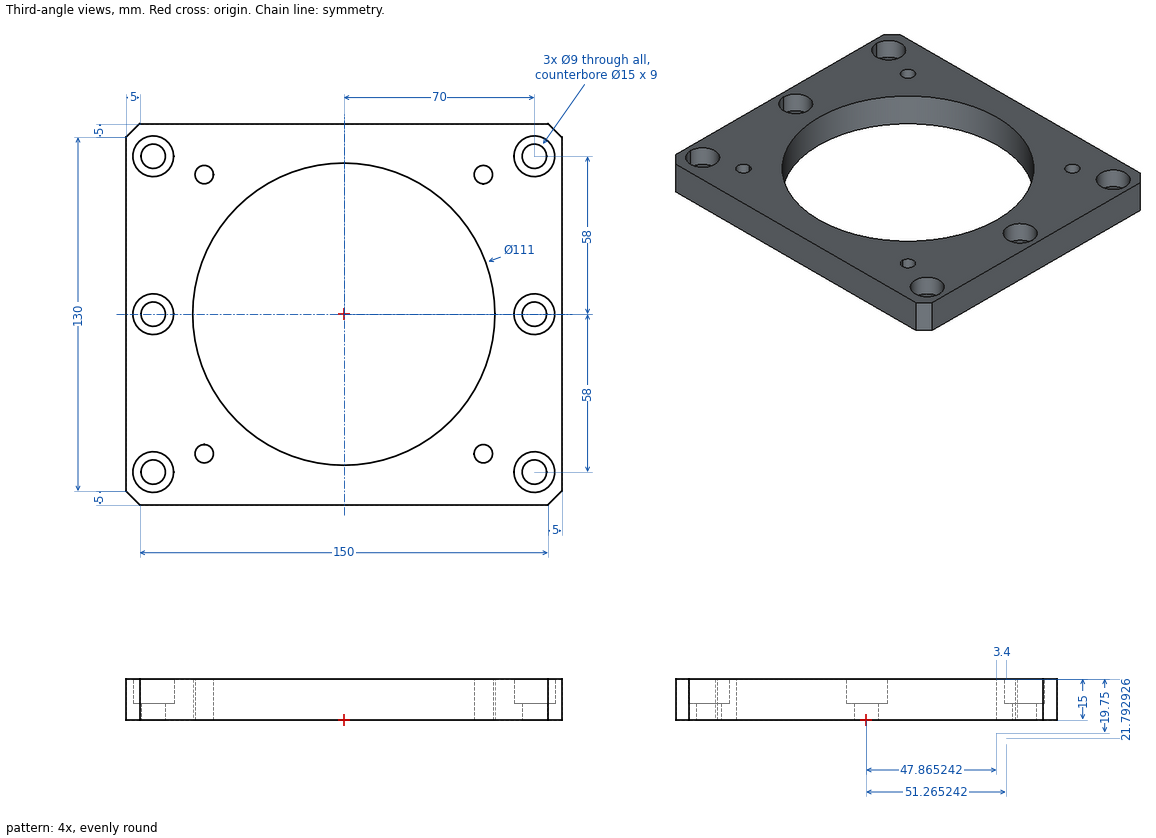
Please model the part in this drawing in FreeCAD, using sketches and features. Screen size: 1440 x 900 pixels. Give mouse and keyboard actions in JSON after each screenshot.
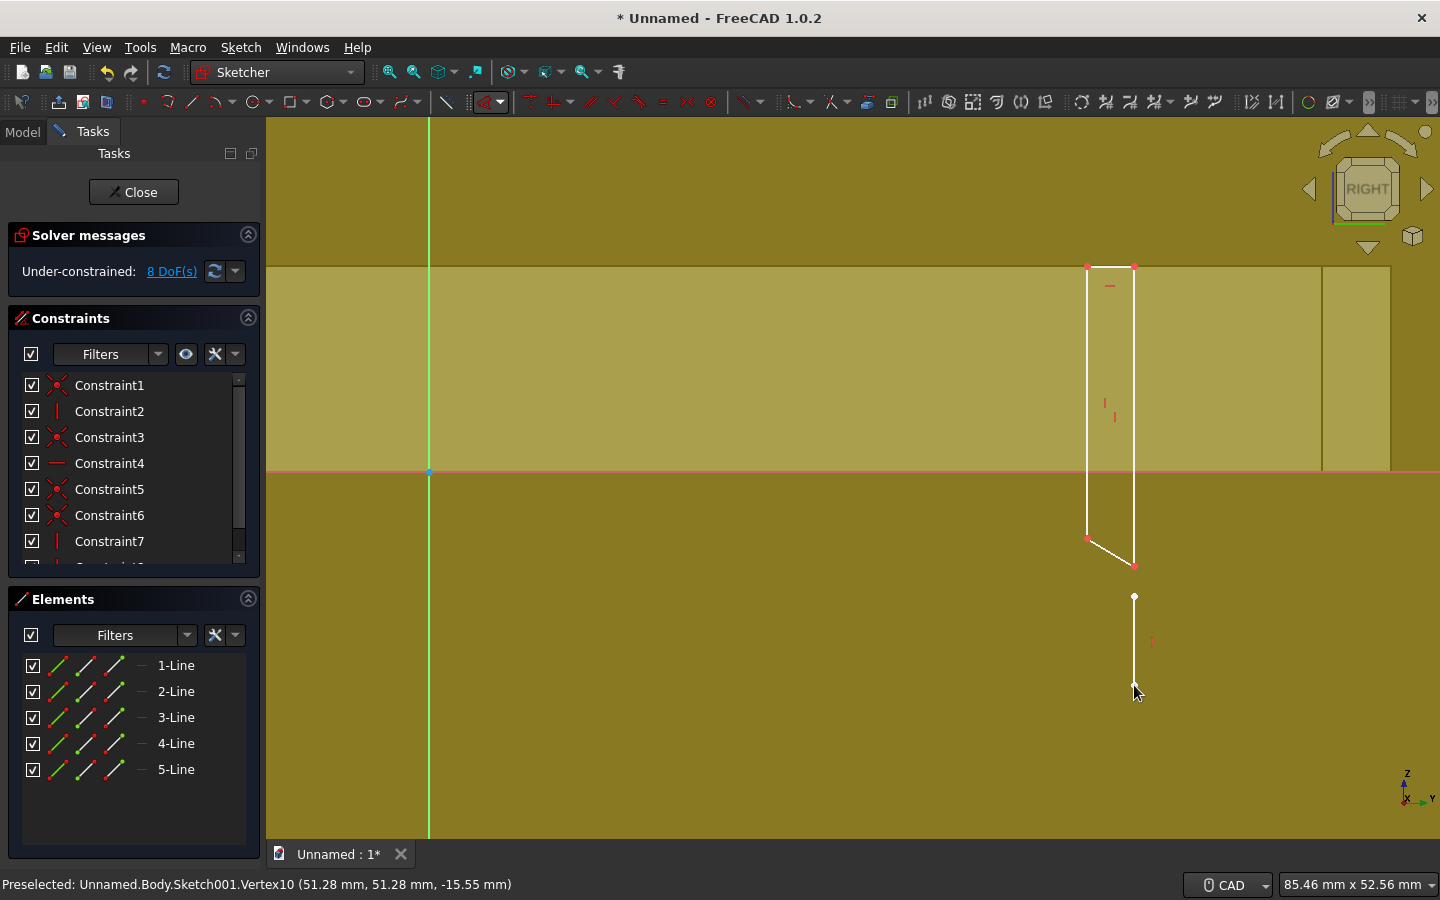
{"action": "left_click", "coordinate": [1134, 624]}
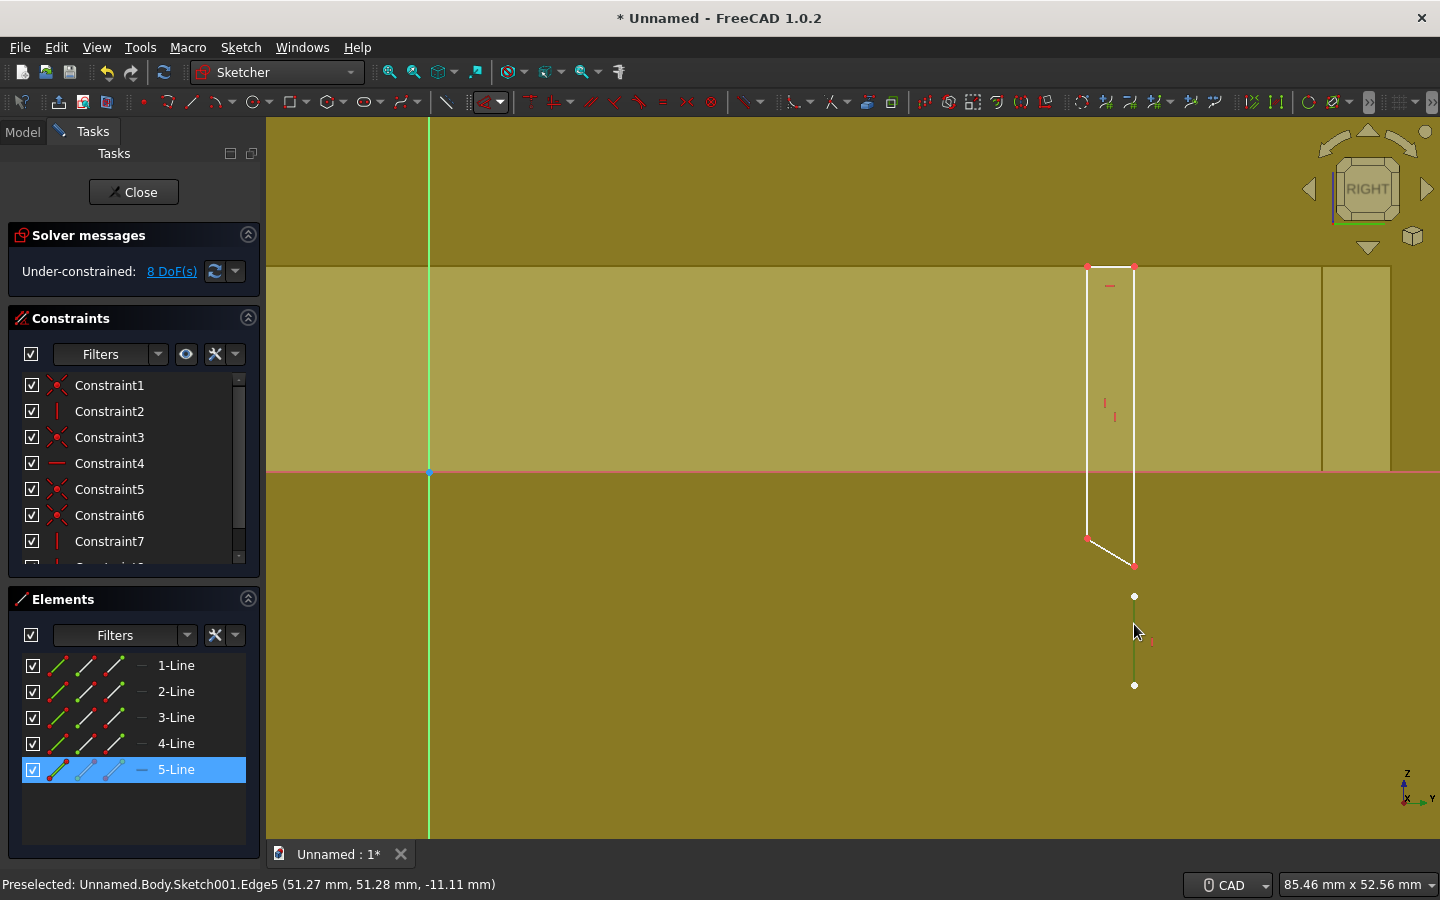
{"action": "left_click", "coordinate": [448, 102]}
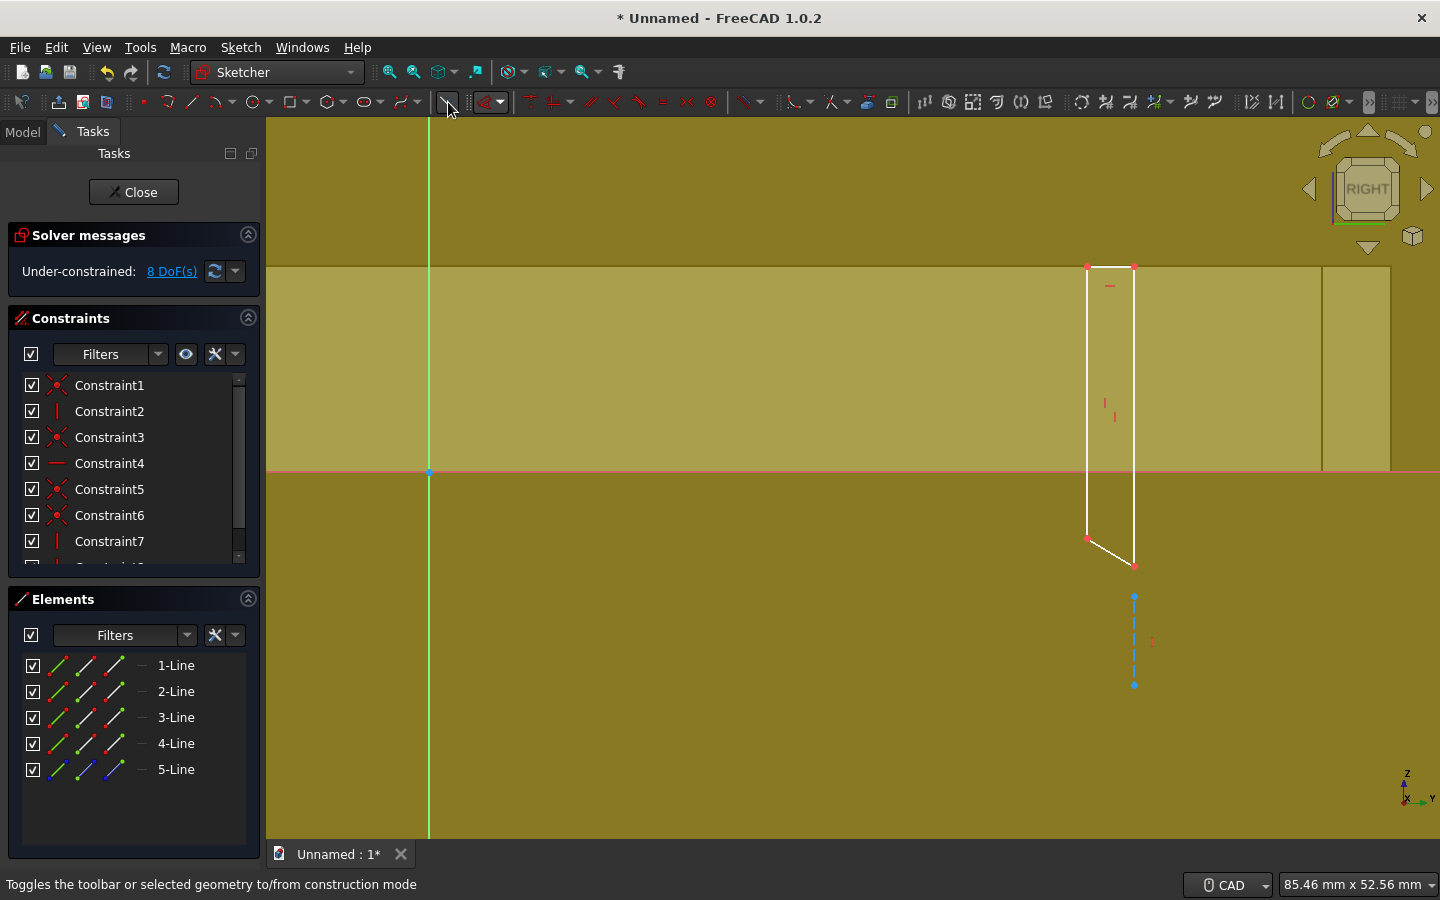
{"action": "left_click", "coordinate": [1120, 267]}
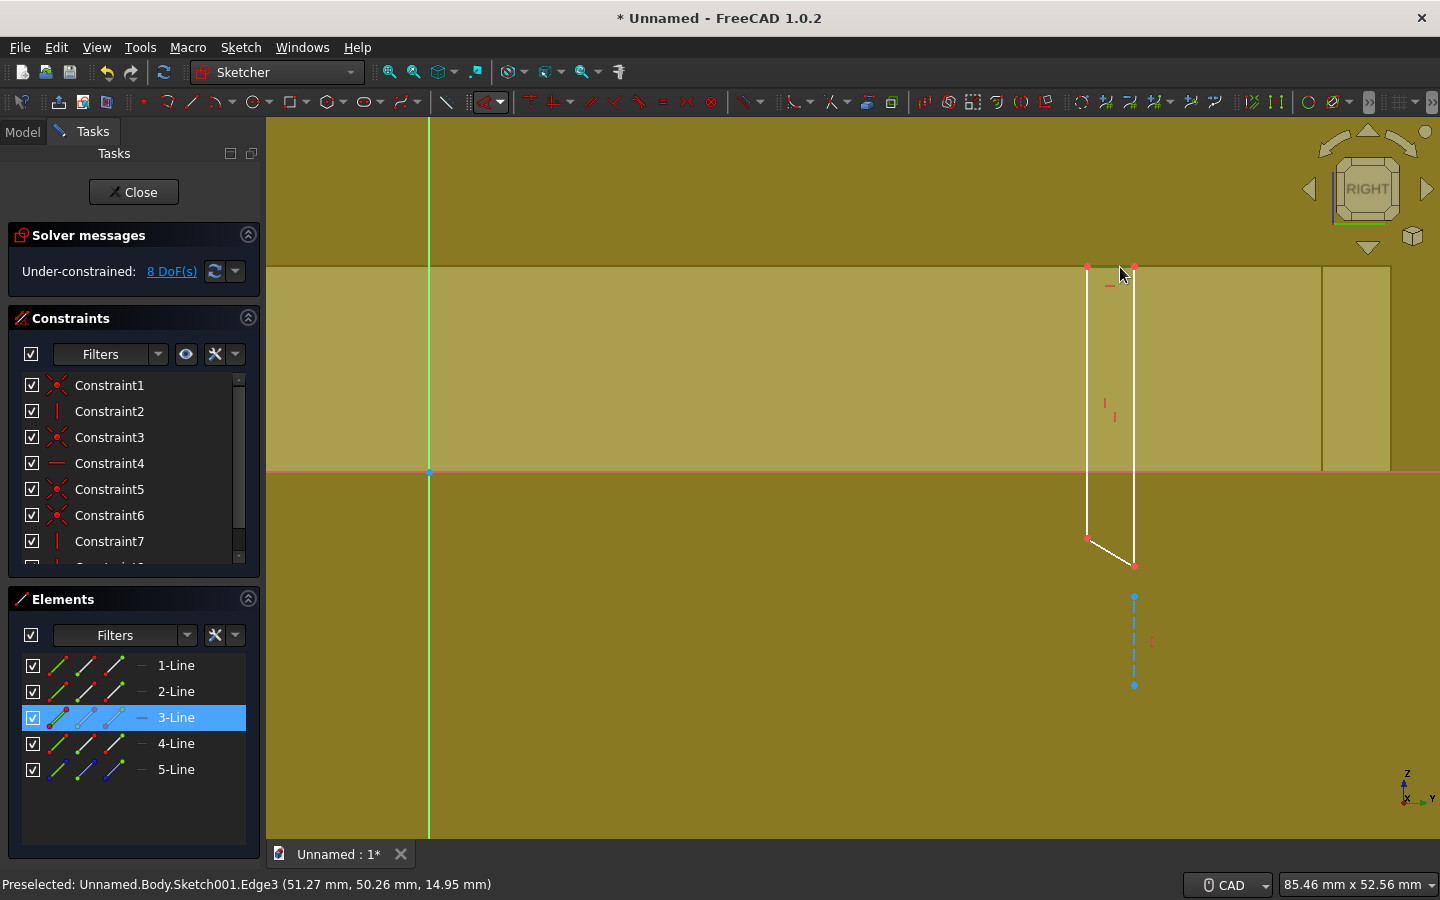
{"action": "key", "text": "l"}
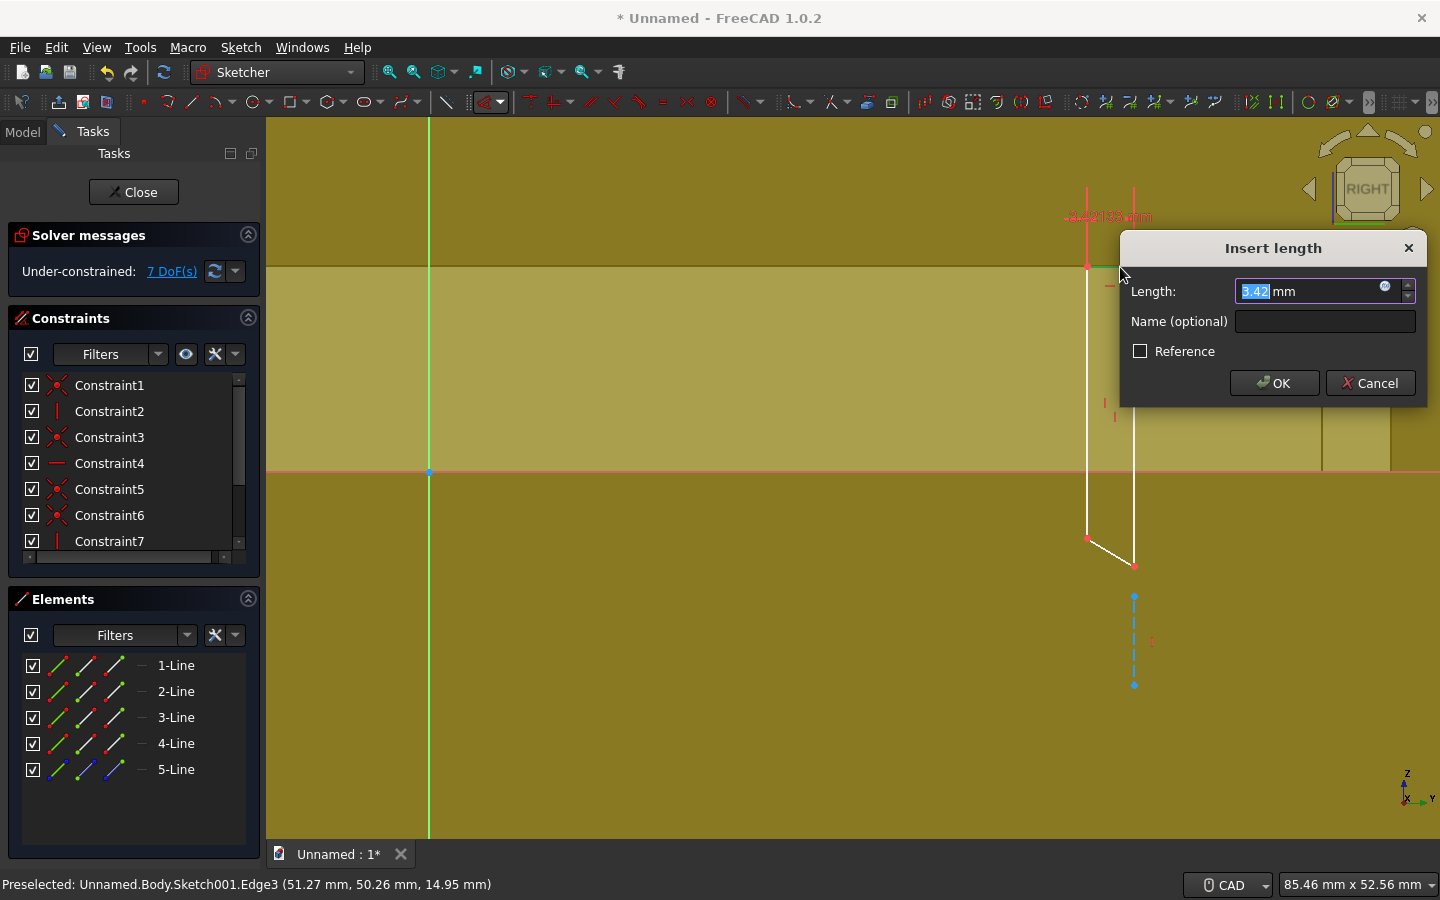
{"action": "type", "text": "3.4"}
{"action": "key", "text": "Return"}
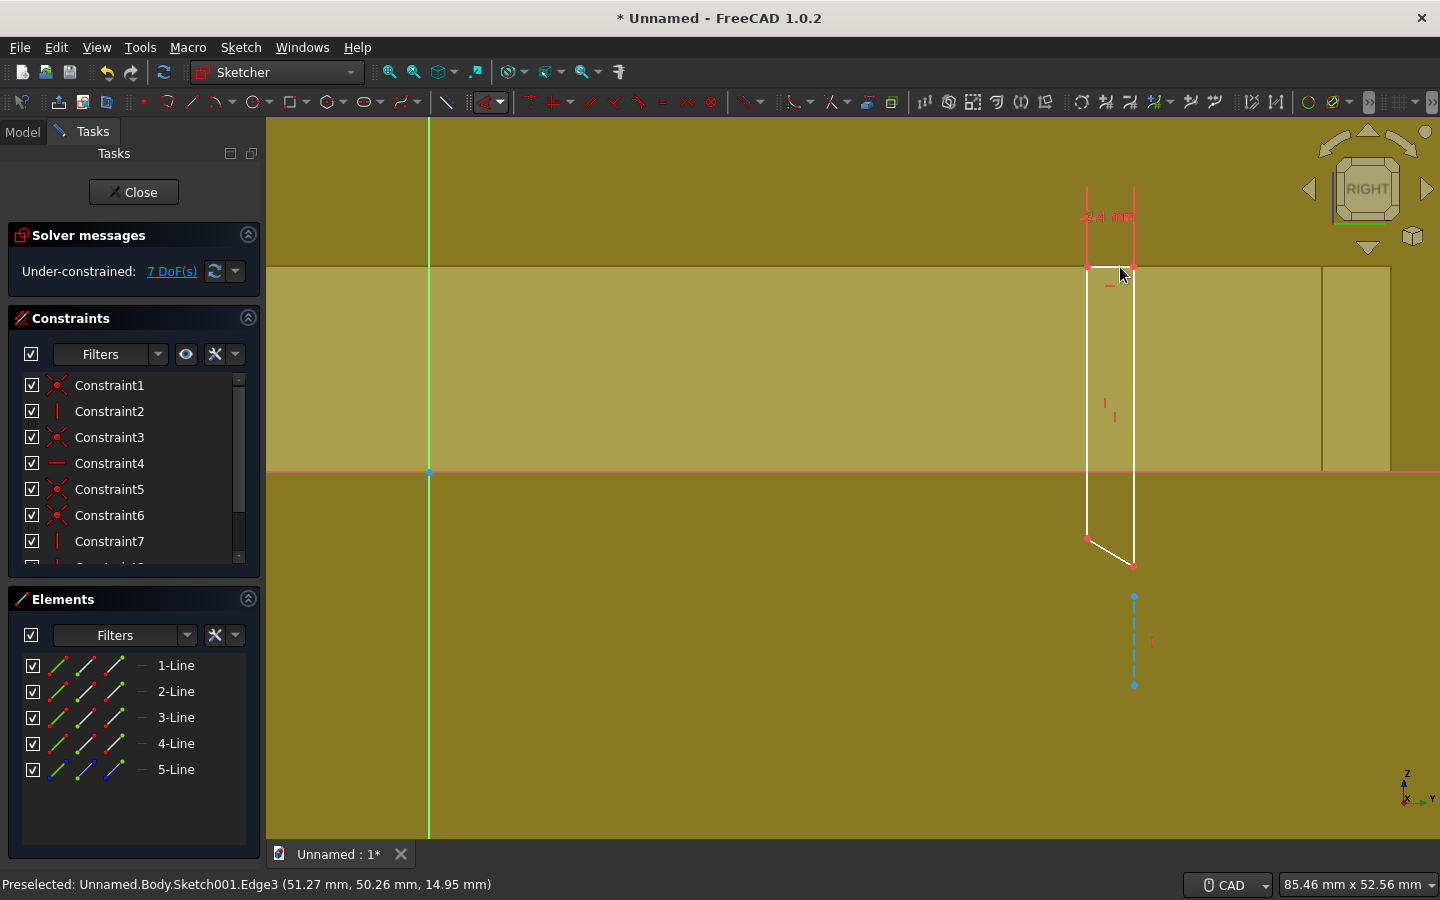
{"action": "left_click", "coordinate": [1134, 267]}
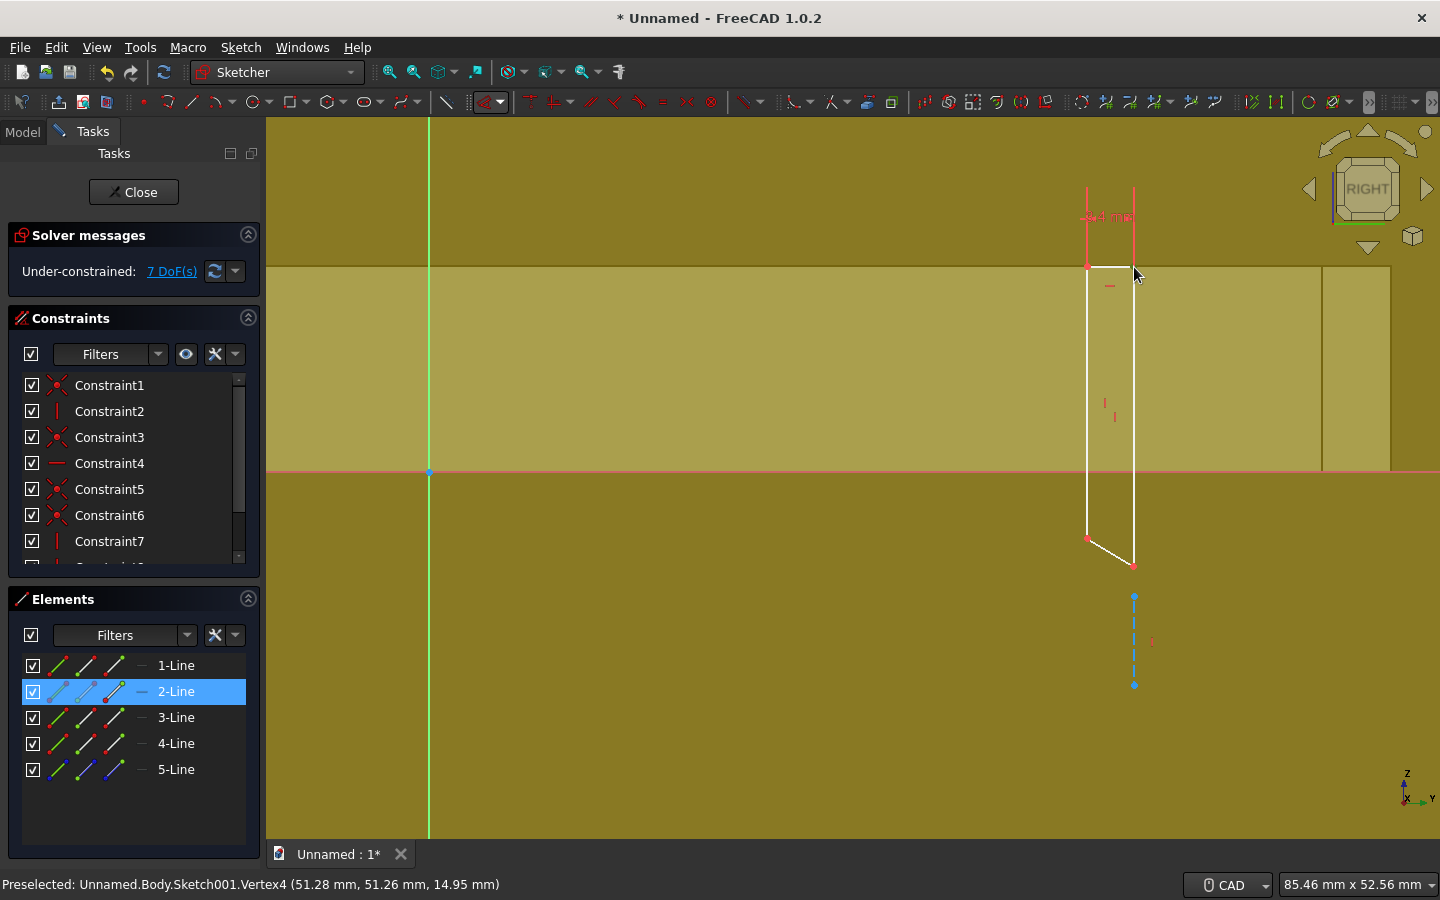
{"action": "left_click", "coordinate": [502, 102]}